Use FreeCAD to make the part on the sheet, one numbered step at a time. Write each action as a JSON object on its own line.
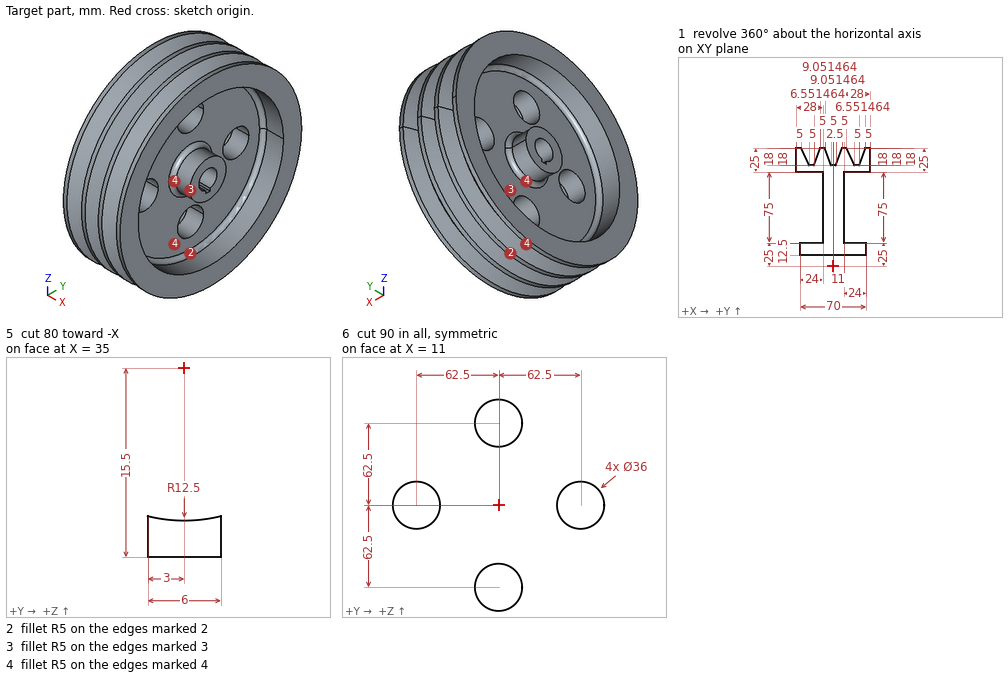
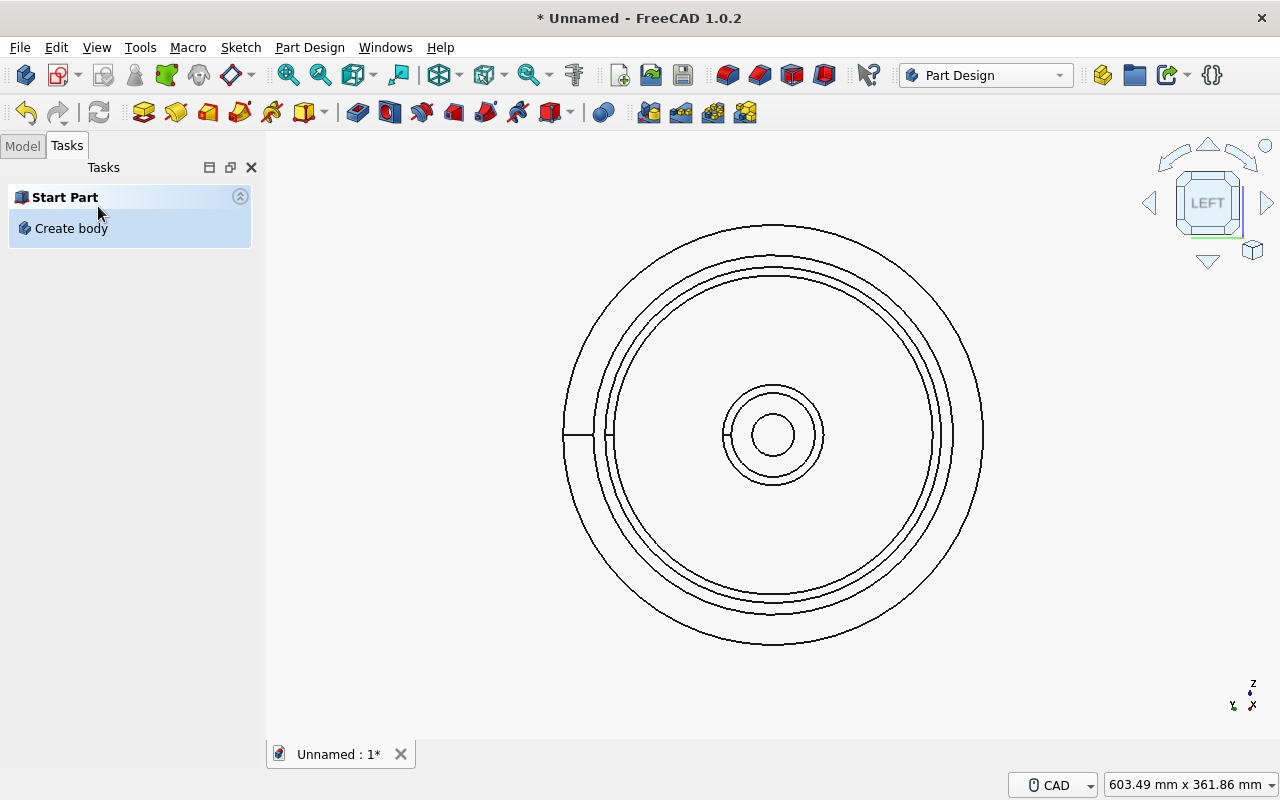
{"action": "key", "text": "0"}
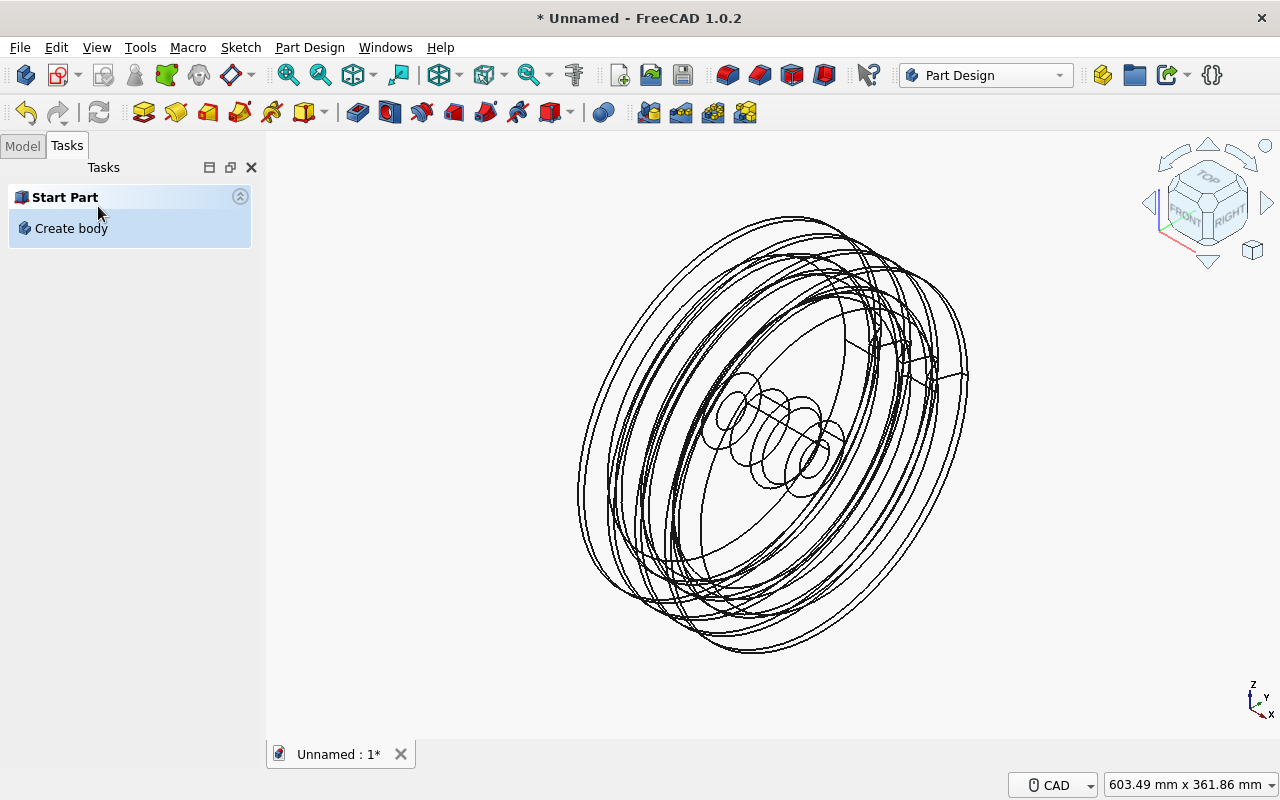
{"action": "left_click", "coordinate": [730, 444]}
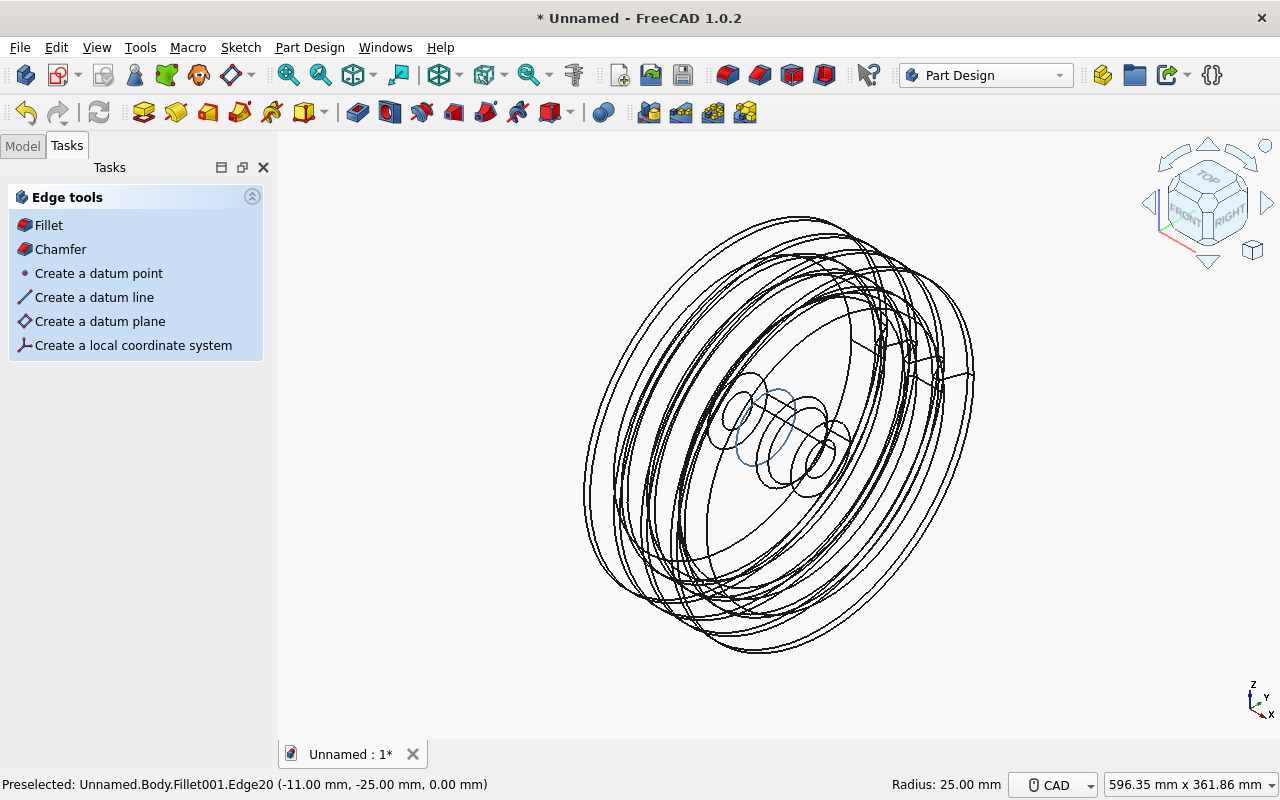
{"action": "left_click", "coordinate": [729, 578], "text": "ctrl"}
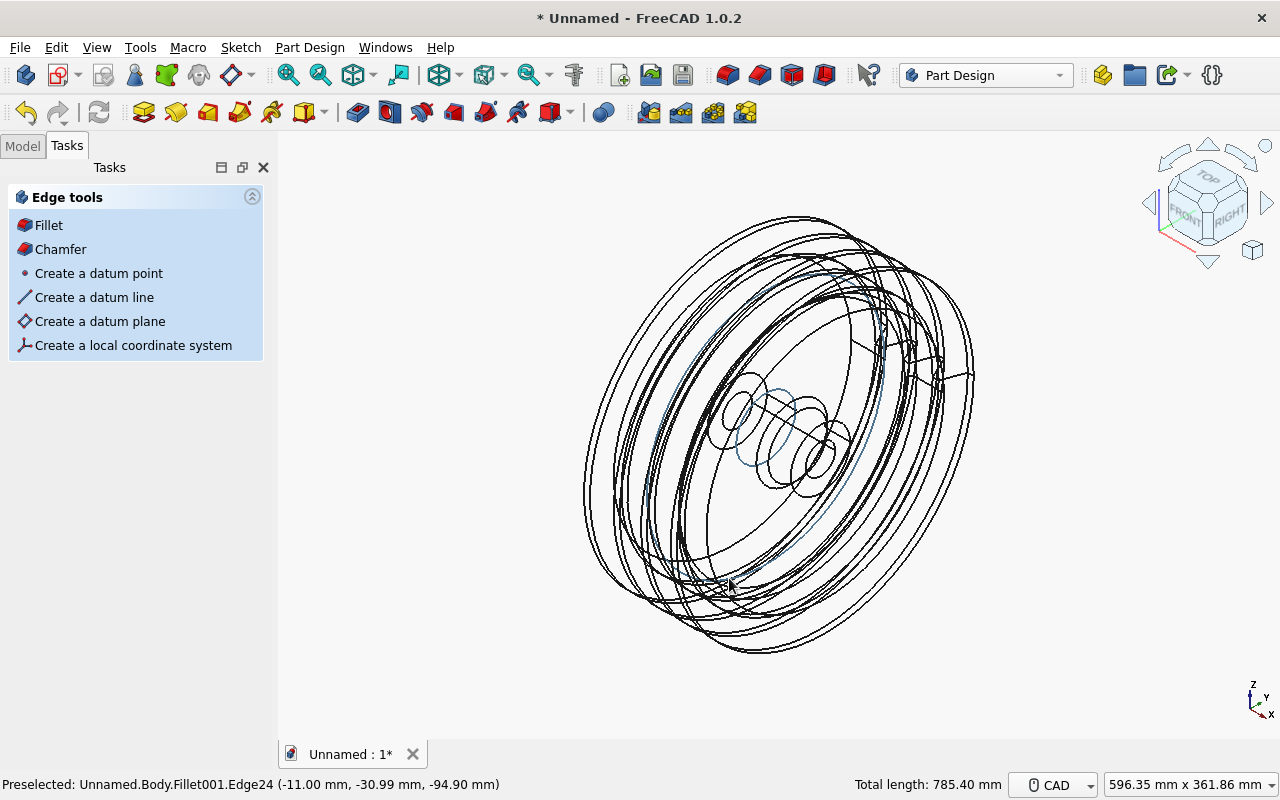
{"action": "key", "text": "v 1"}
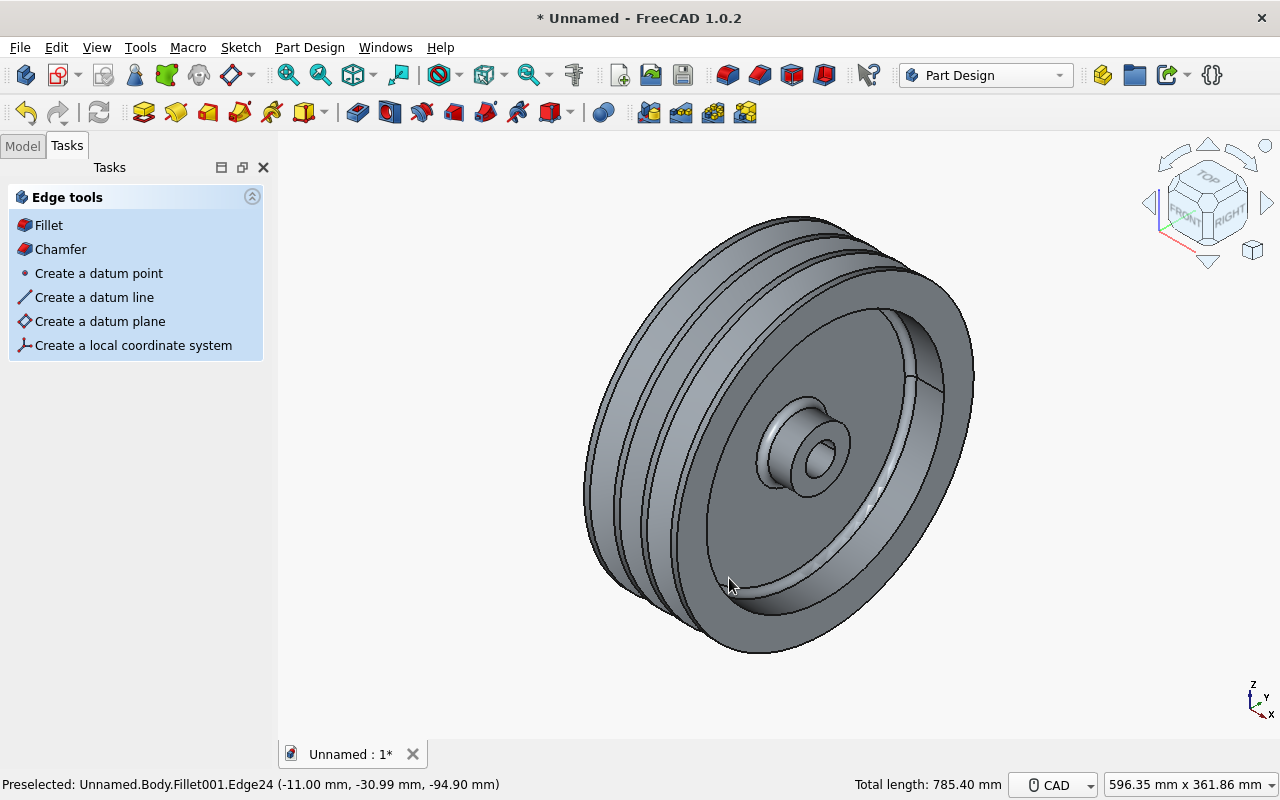
{"action": "left_click", "coordinate": [728, 76]}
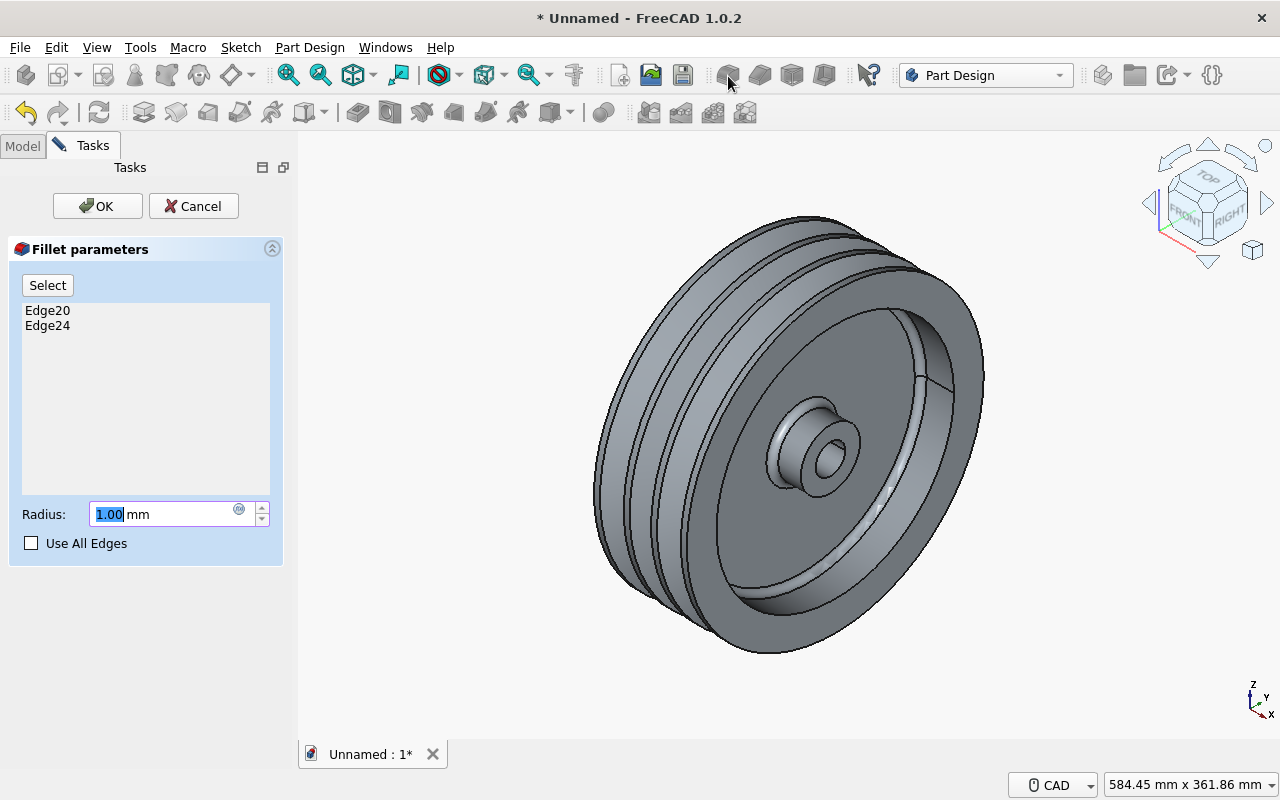
{"action": "type", "text": "5"}
{"action": "key", "text": "Tab"}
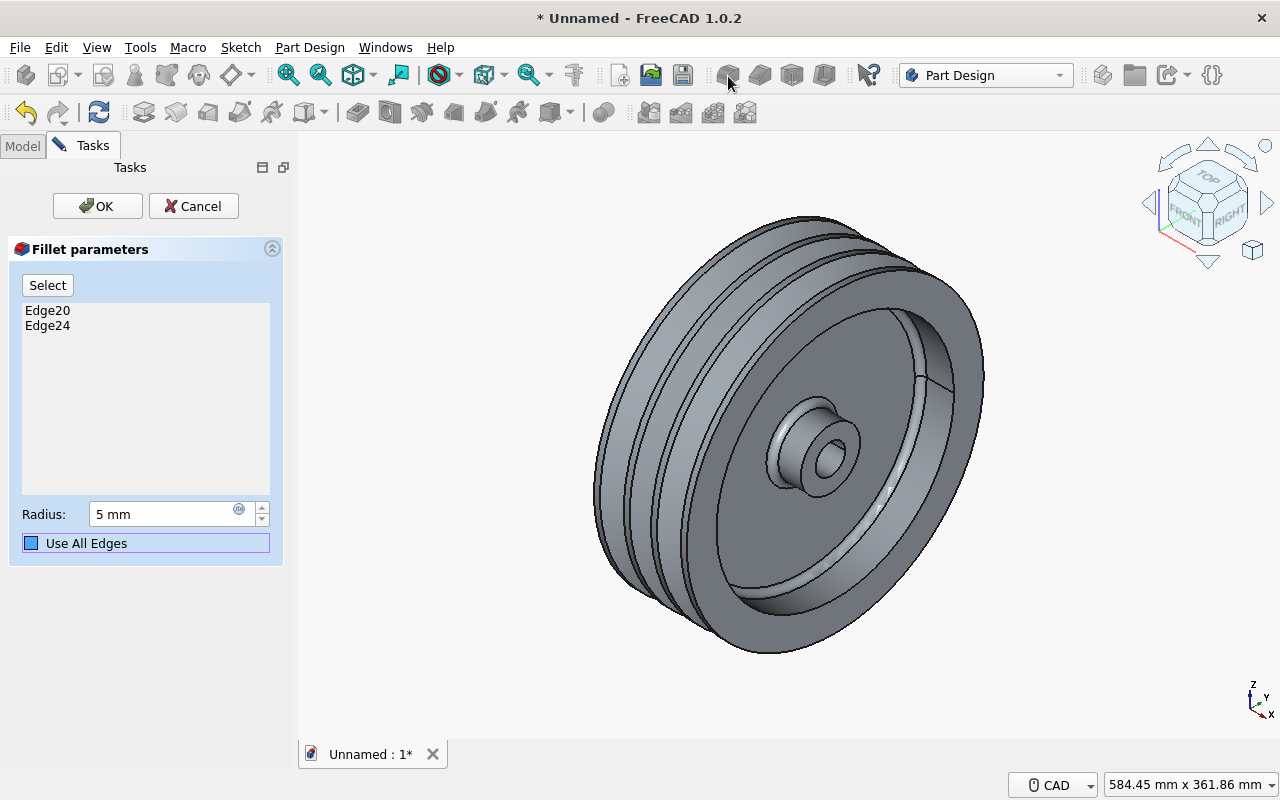
{"action": "left_click", "coordinate": [98, 206]}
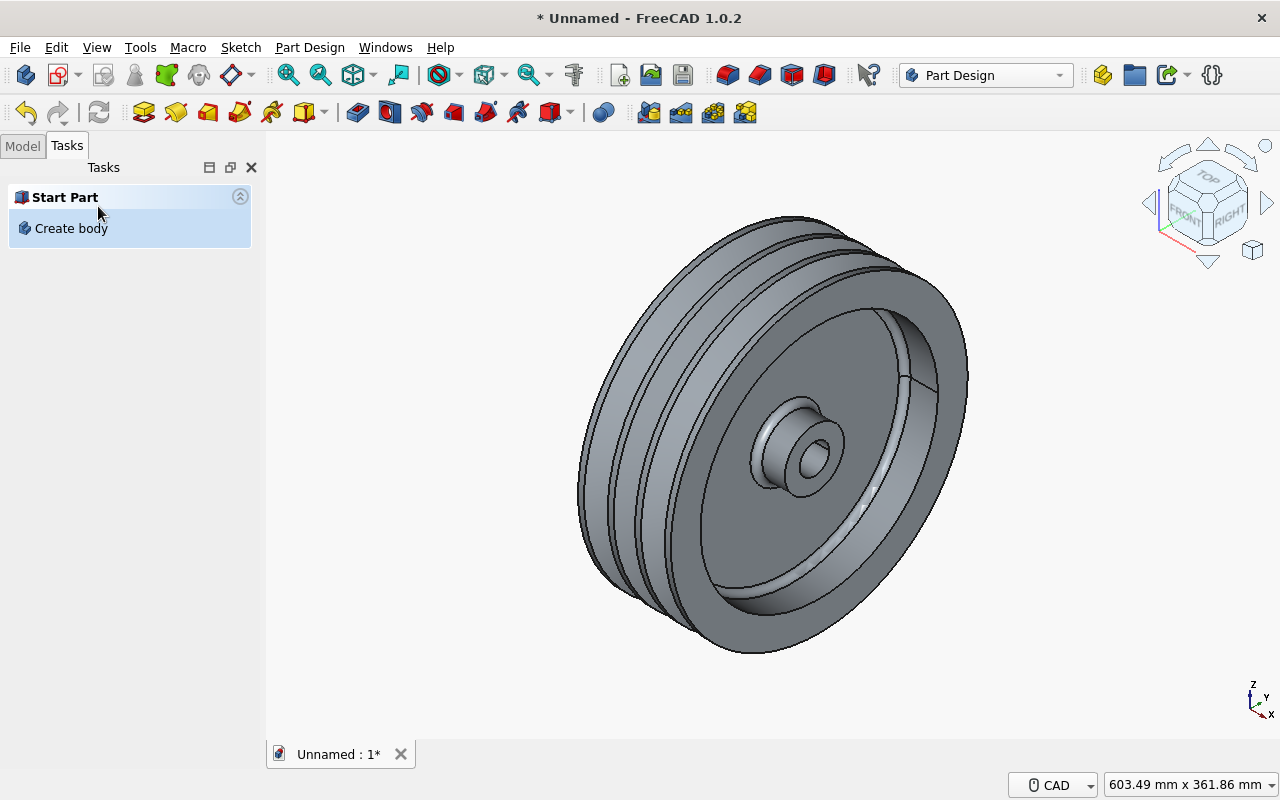
{"action": "left_click", "coordinate": [840, 443]}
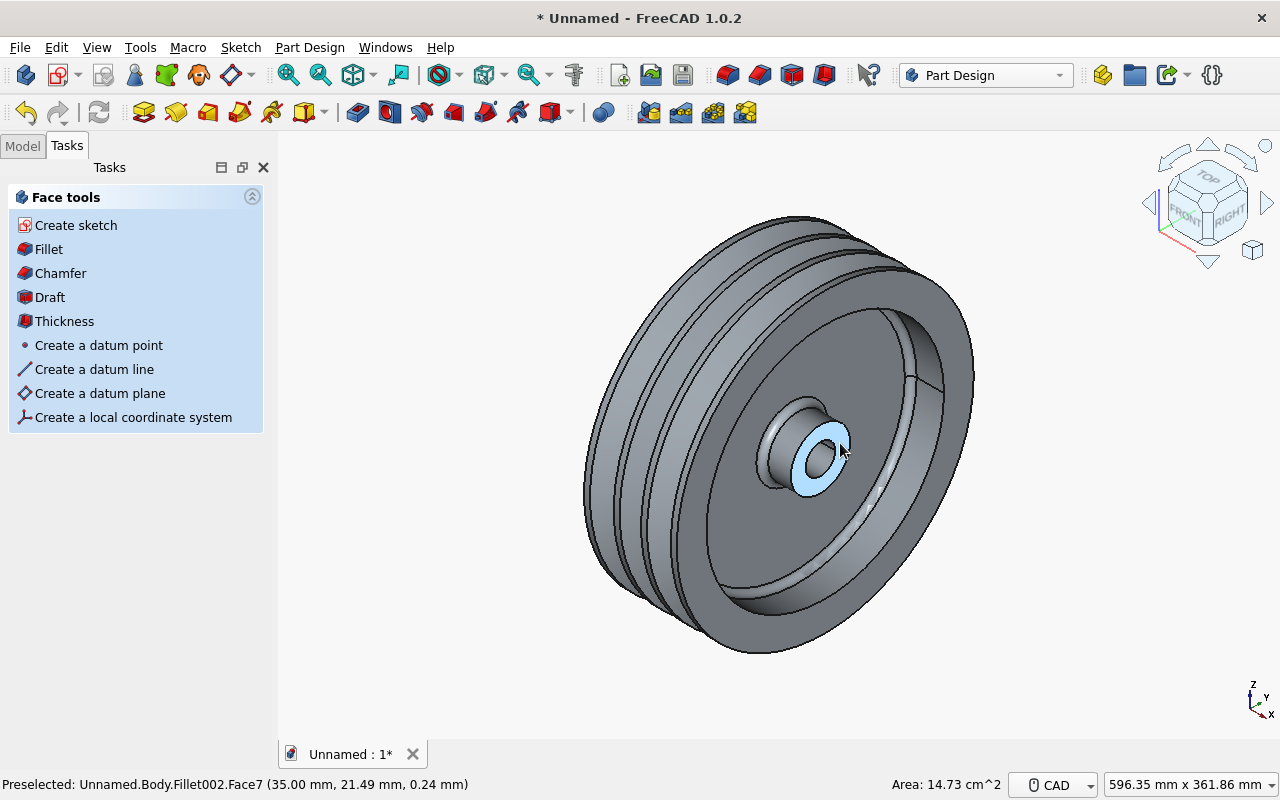
{"action": "left_click", "coordinate": [58, 76]}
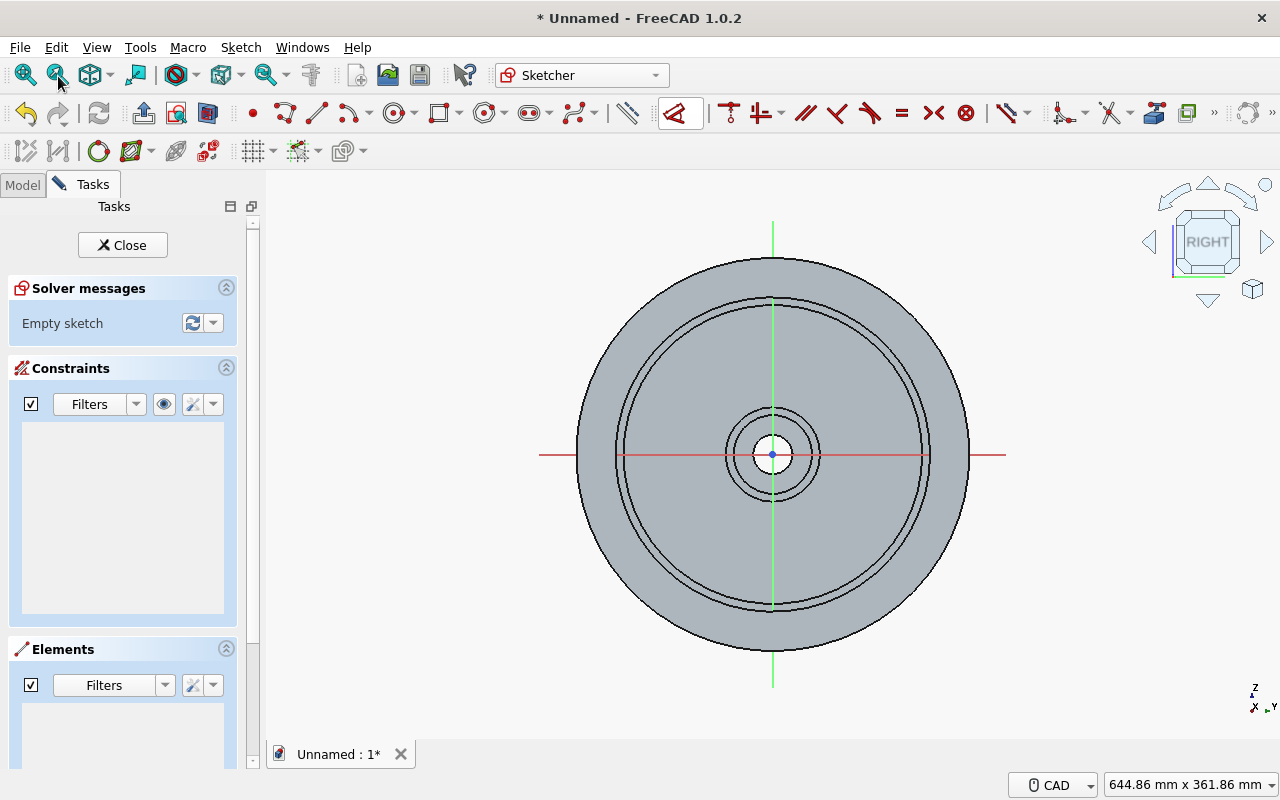
{"action": "scroll", "coordinate": [776, 477], "scroll_direction": "up", "scroll_amount": 15}